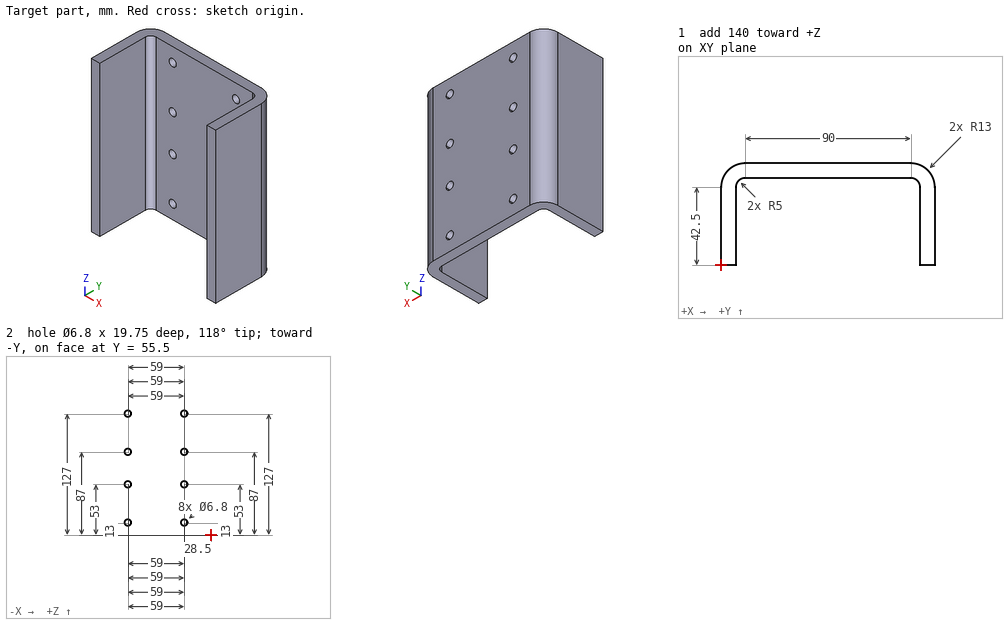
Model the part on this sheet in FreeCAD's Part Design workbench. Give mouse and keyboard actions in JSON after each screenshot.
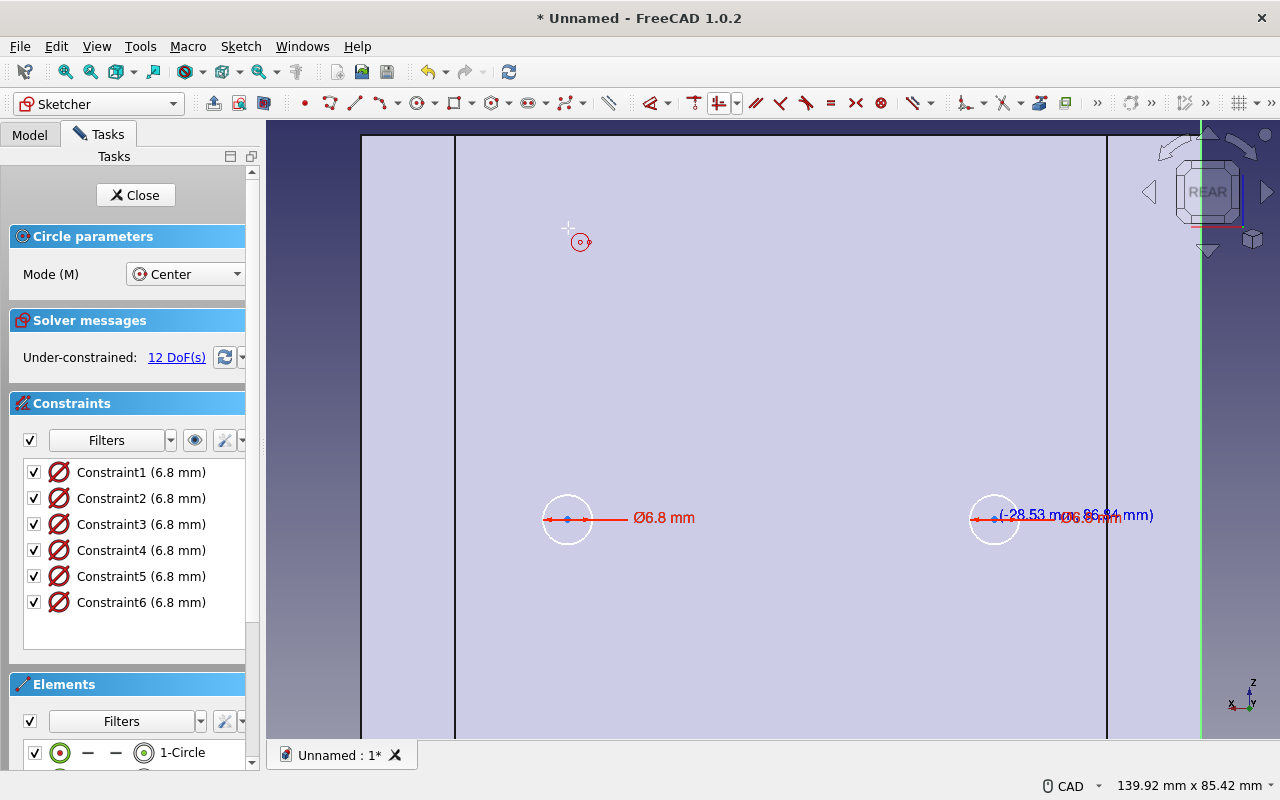
{"action": "left_click", "coordinate": [567, 229]}
{"action": "mouse_move", "coordinate": [585, 211]}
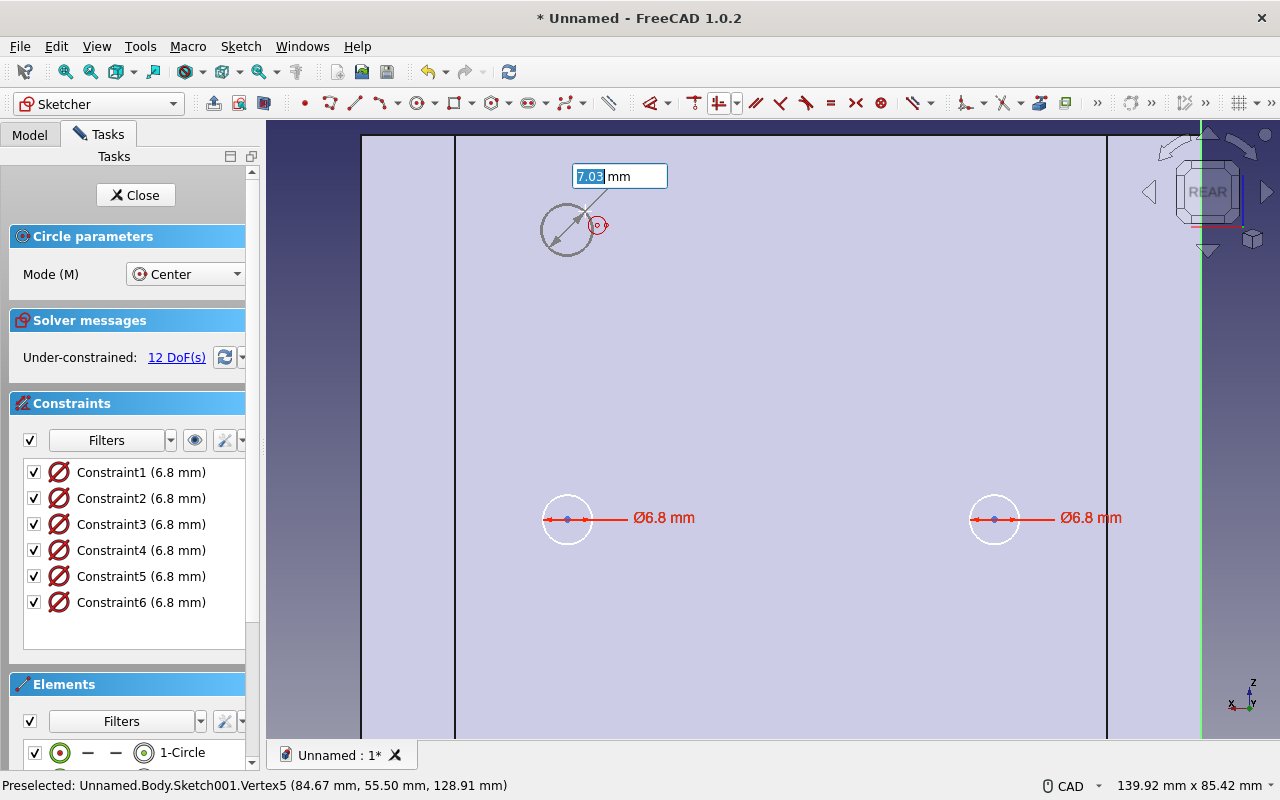
{"action": "type", "text": "6.8"}
{"action": "key", "text": "Return"}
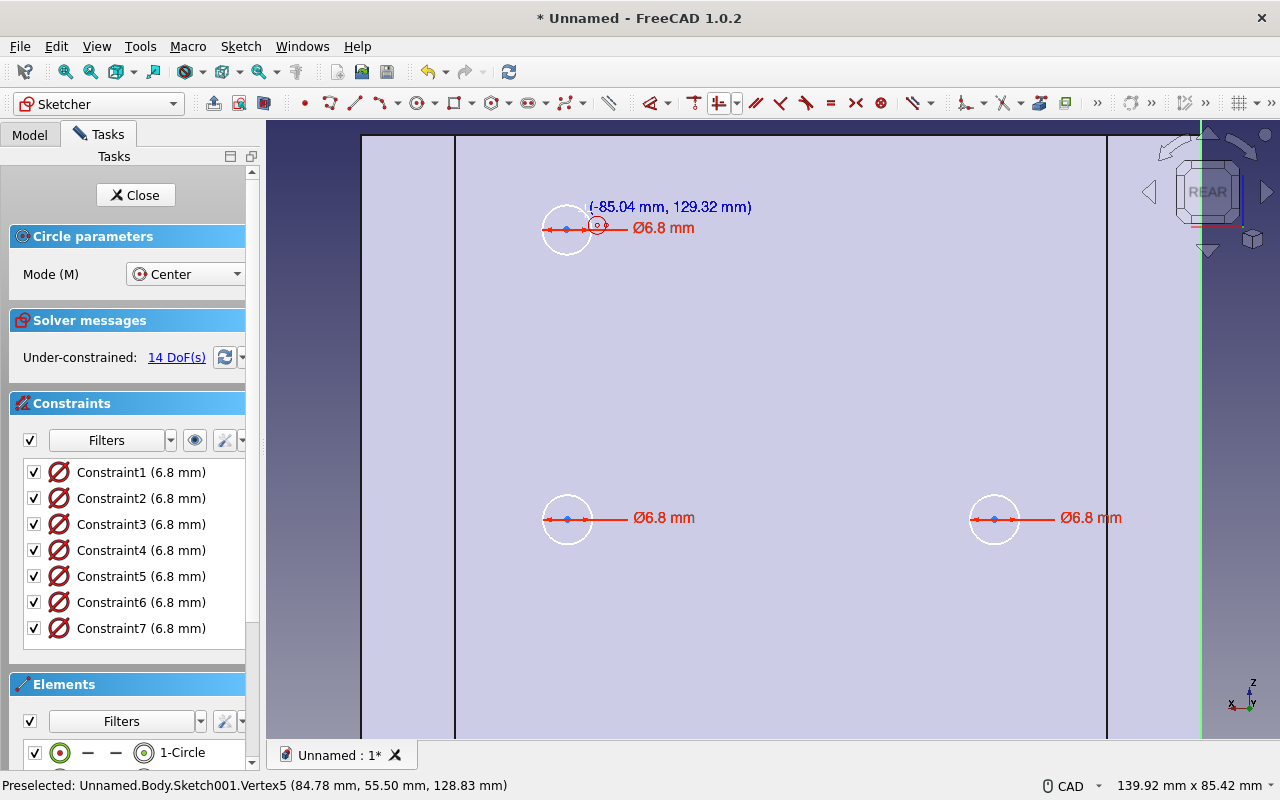
{"action": "left_click", "coordinate": [995, 229]}
{"action": "mouse_move", "coordinate": [1012, 211]}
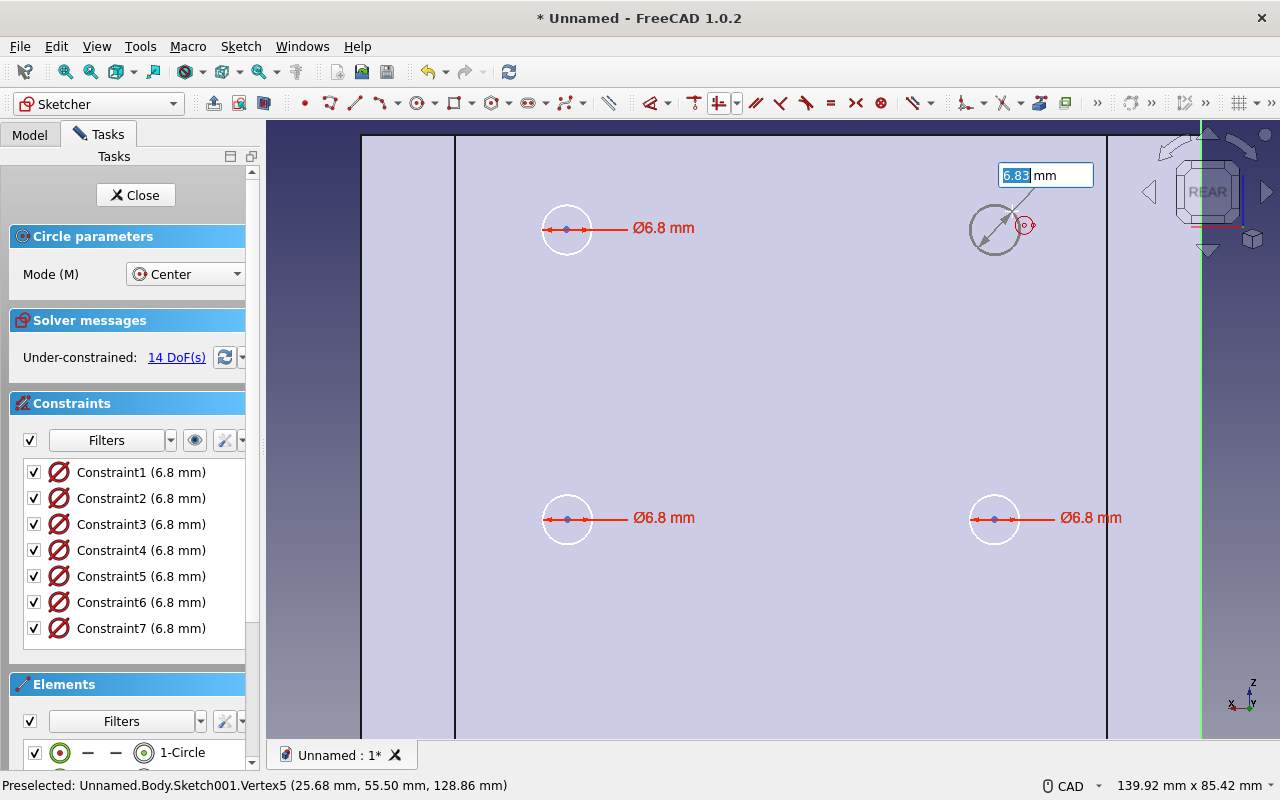
{"action": "type", "text": "6.8"}
{"action": "key", "text": "Return"}
{"action": "key", "text": "Escape"}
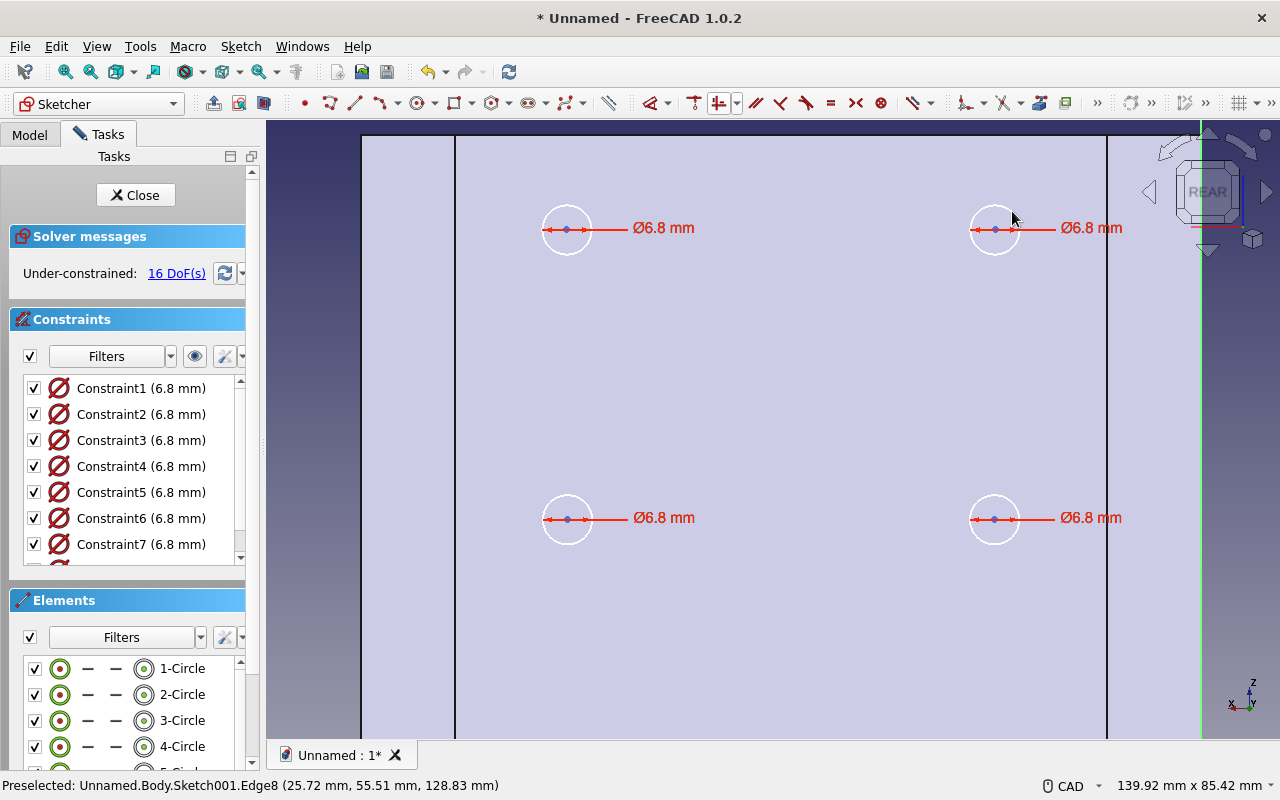
{"action": "key", "text": "d"}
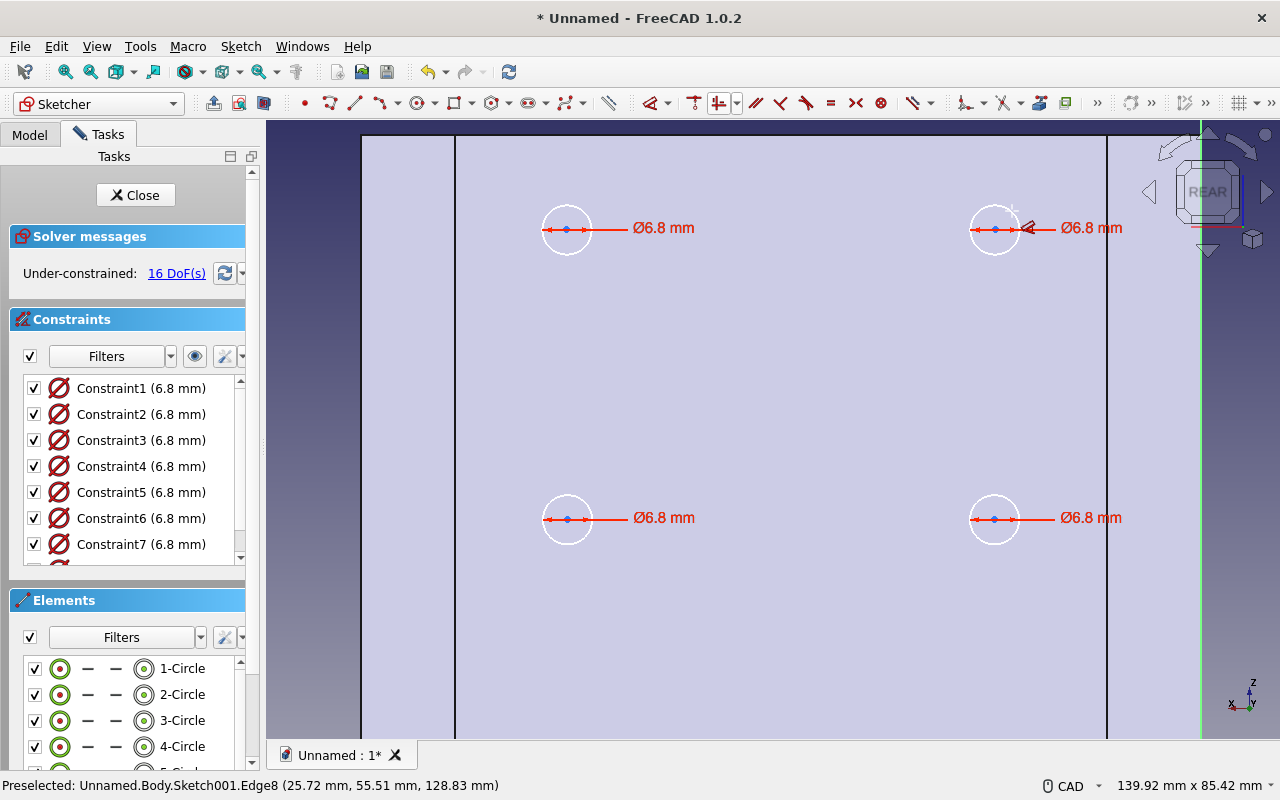
{"action": "scroll", "coordinate": [568, 228], "scroll_direction": "down", "scroll_amount": 4}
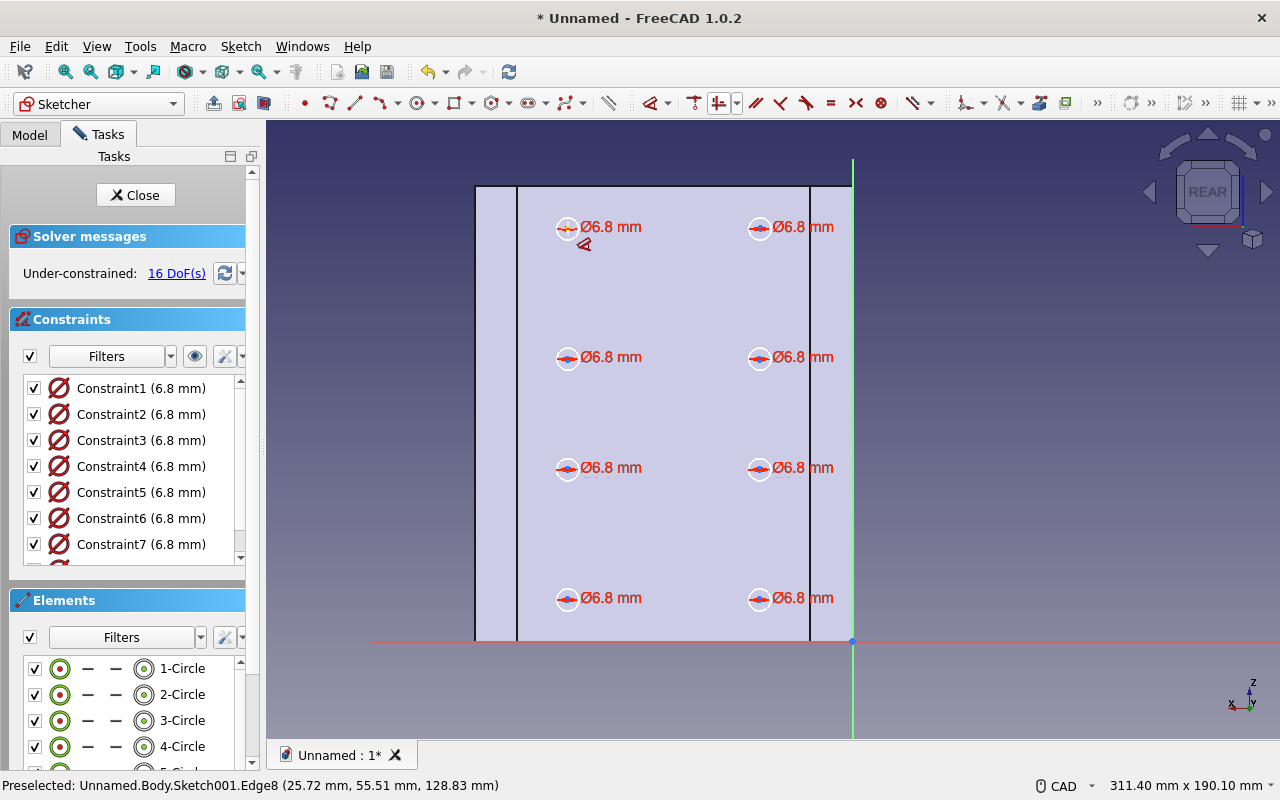
{"action": "left_click", "coordinate": [760, 600]}
{"action": "left_click", "coordinate": [887, 621]}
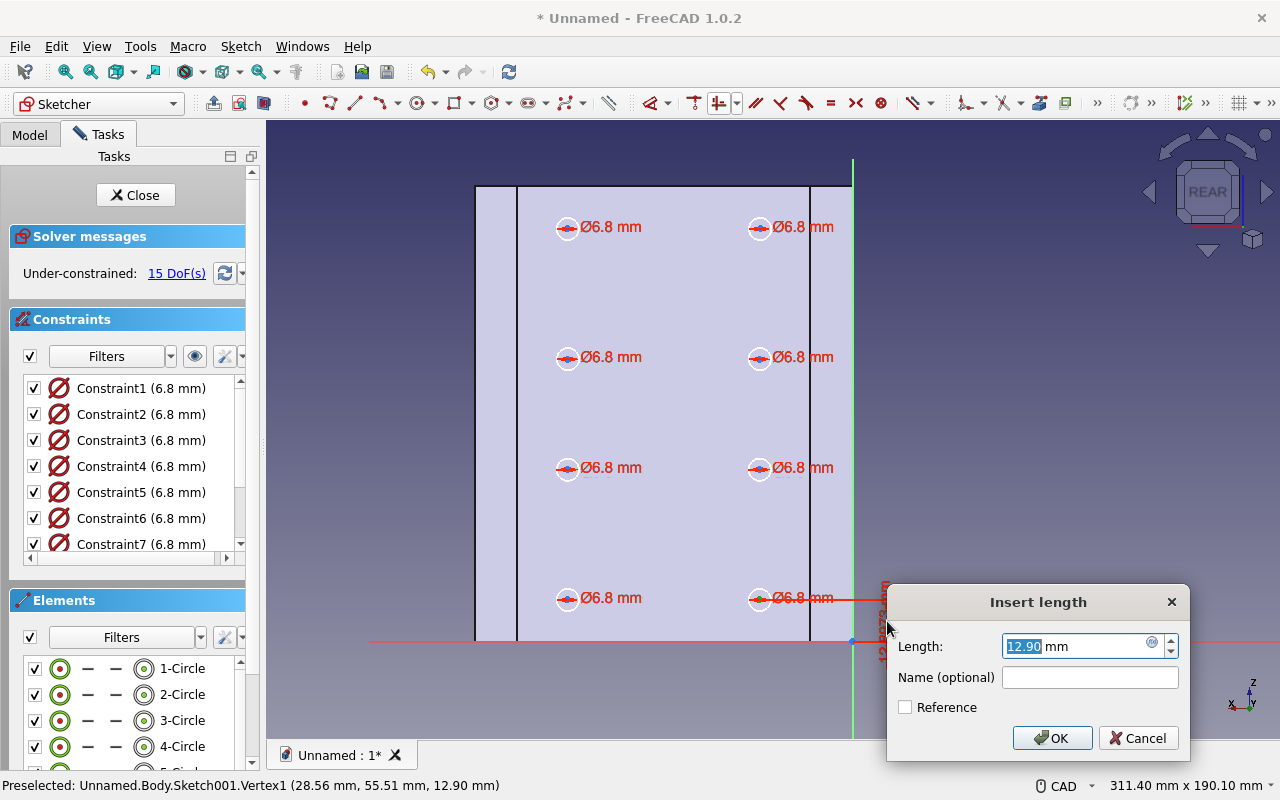
{"action": "type", "text": "13"}
{"action": "key", "text": "Return"}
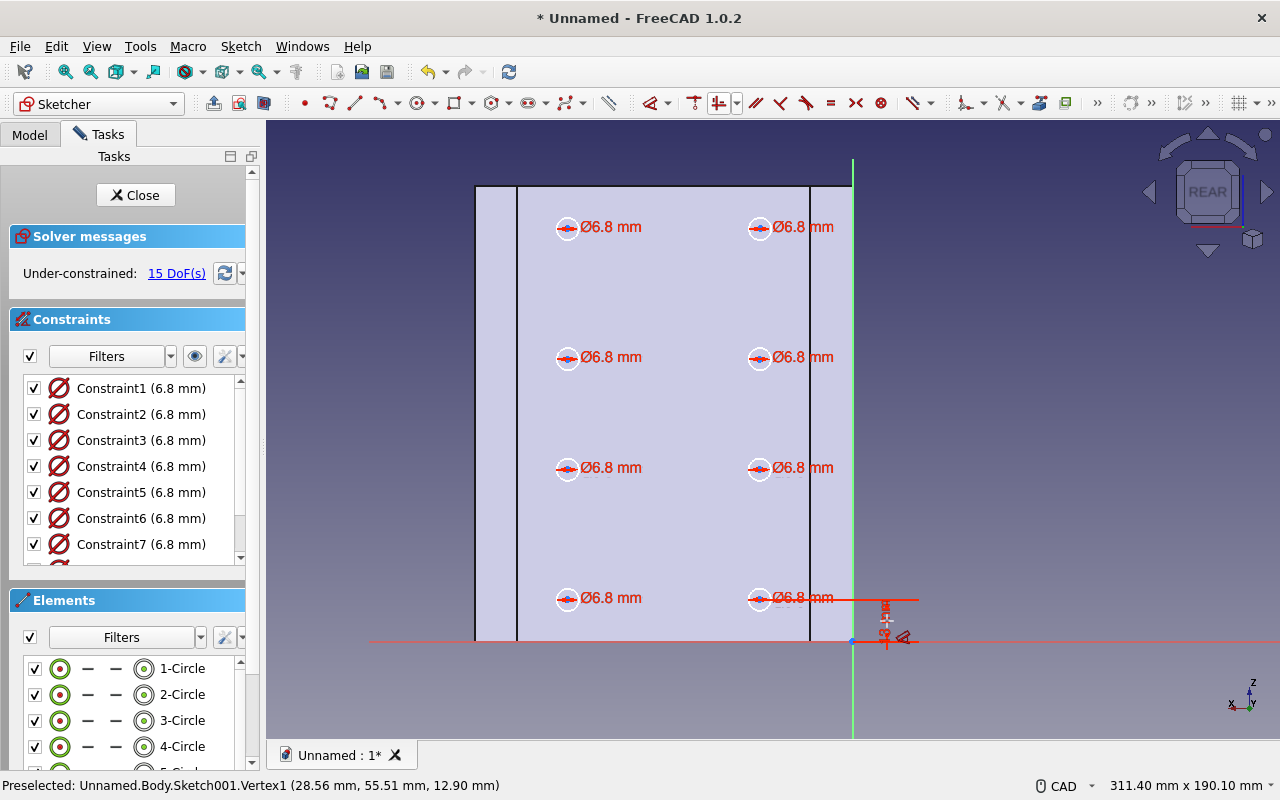
{"action": "left_click", "coordinate": [568, 600]}
{"action": "left_click", "coordinate": [534, 621]}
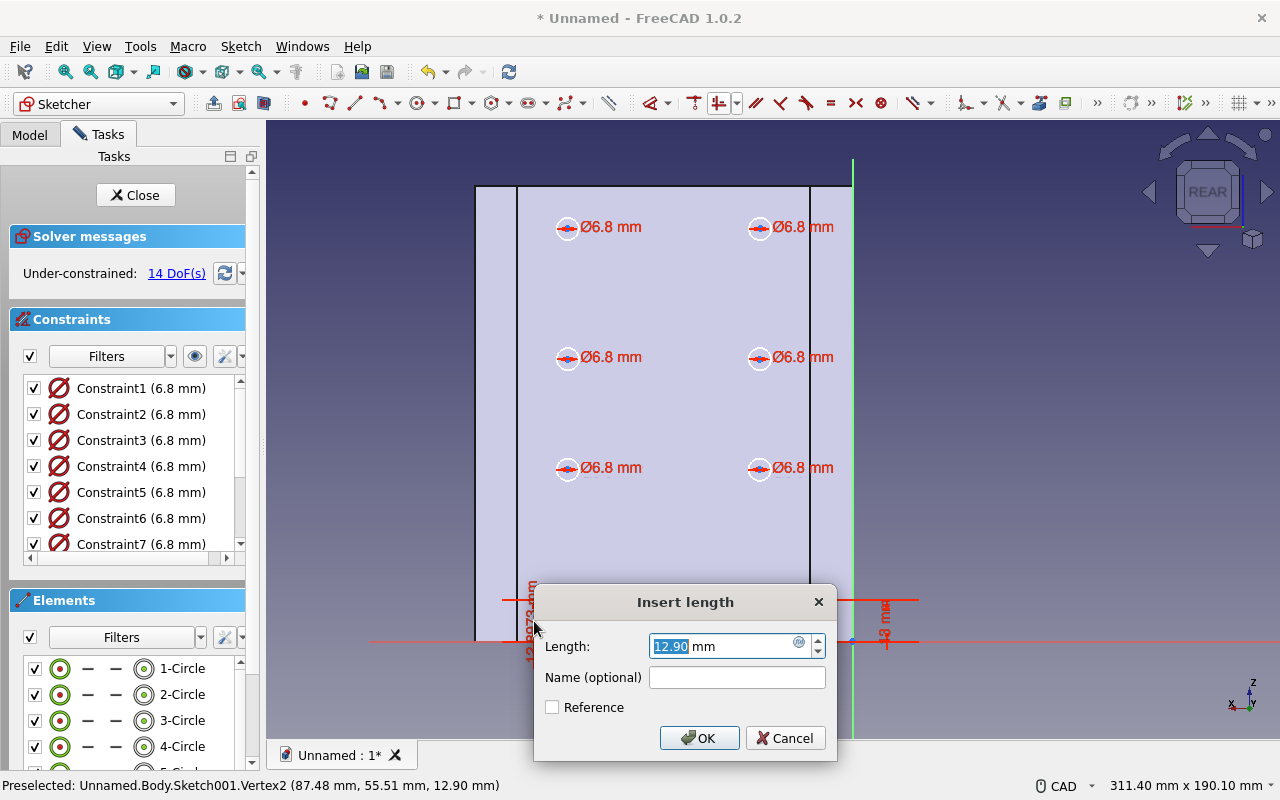
{"action": "type", "text": "13"}
{"action": "key", "text": "Return"}